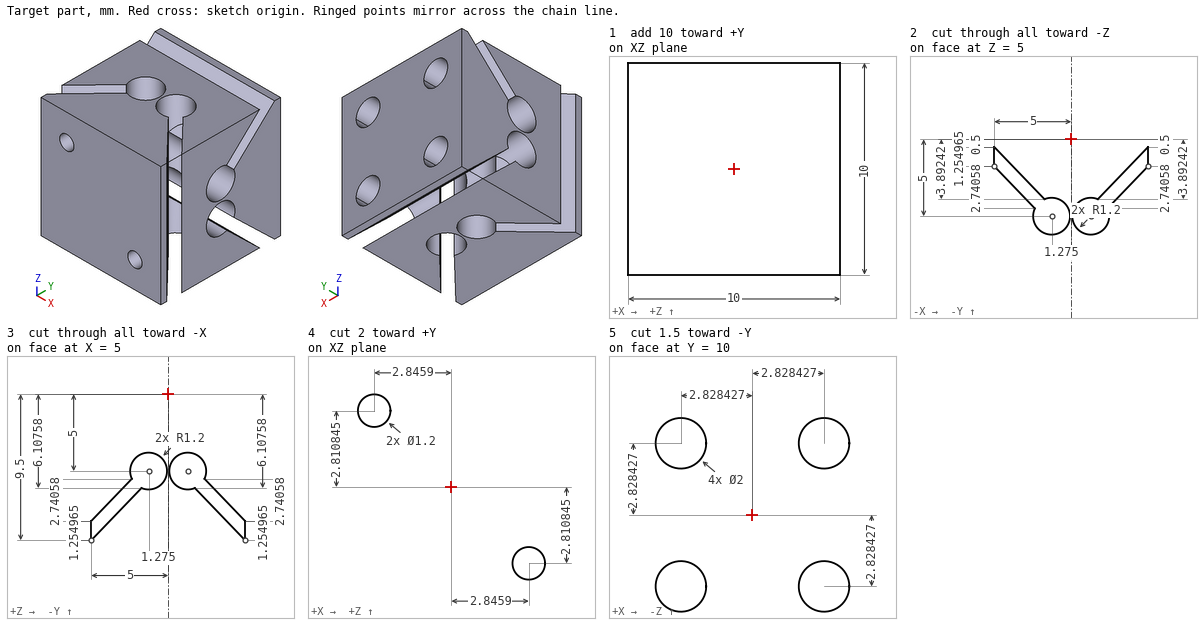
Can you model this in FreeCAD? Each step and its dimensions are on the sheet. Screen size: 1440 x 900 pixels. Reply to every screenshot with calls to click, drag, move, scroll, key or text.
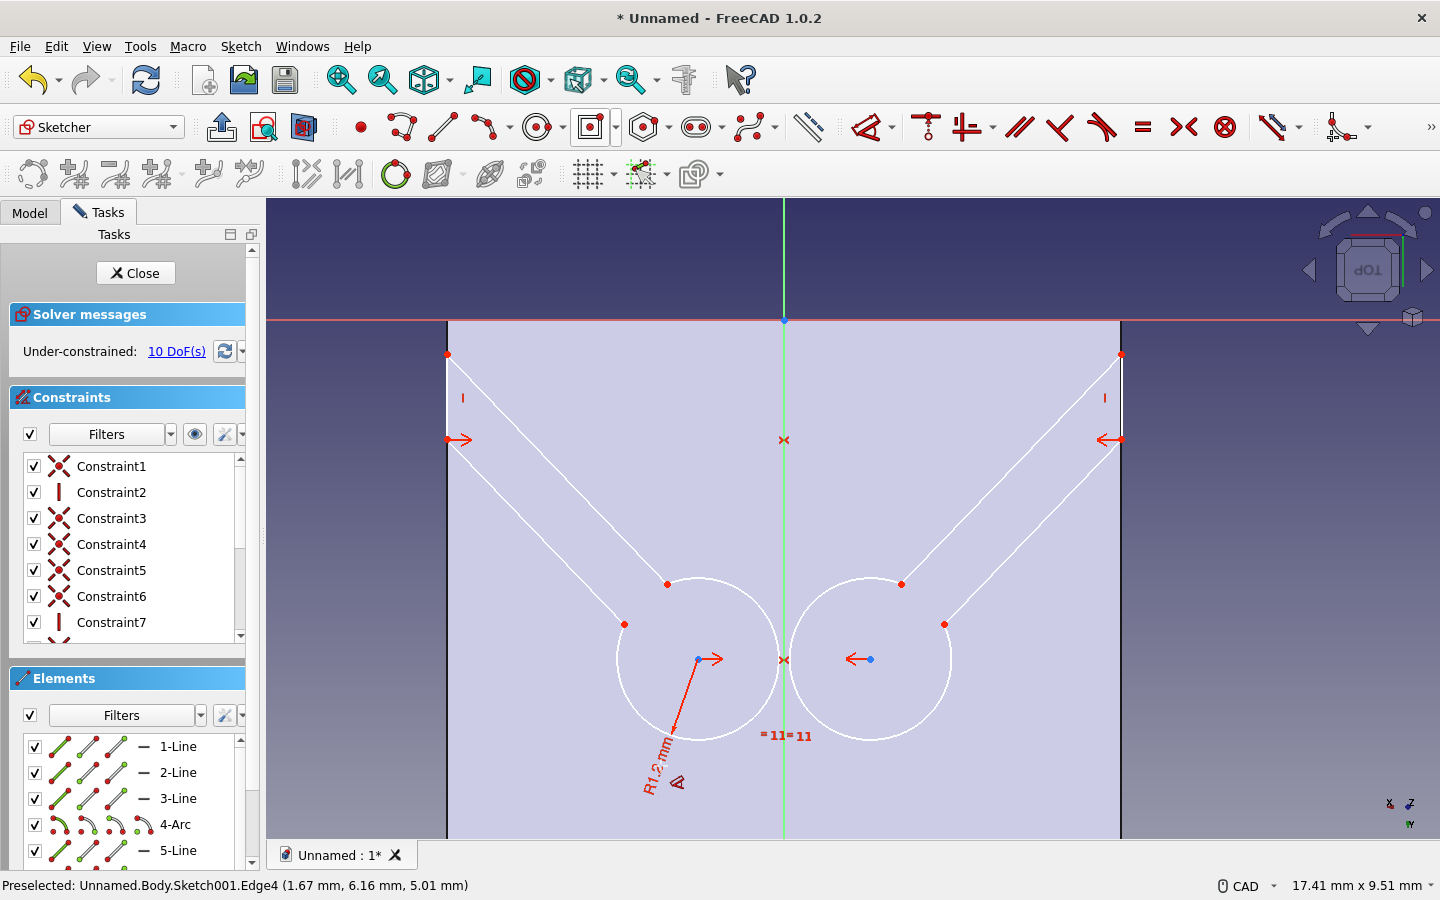
click(447, 355)
click(616, 286)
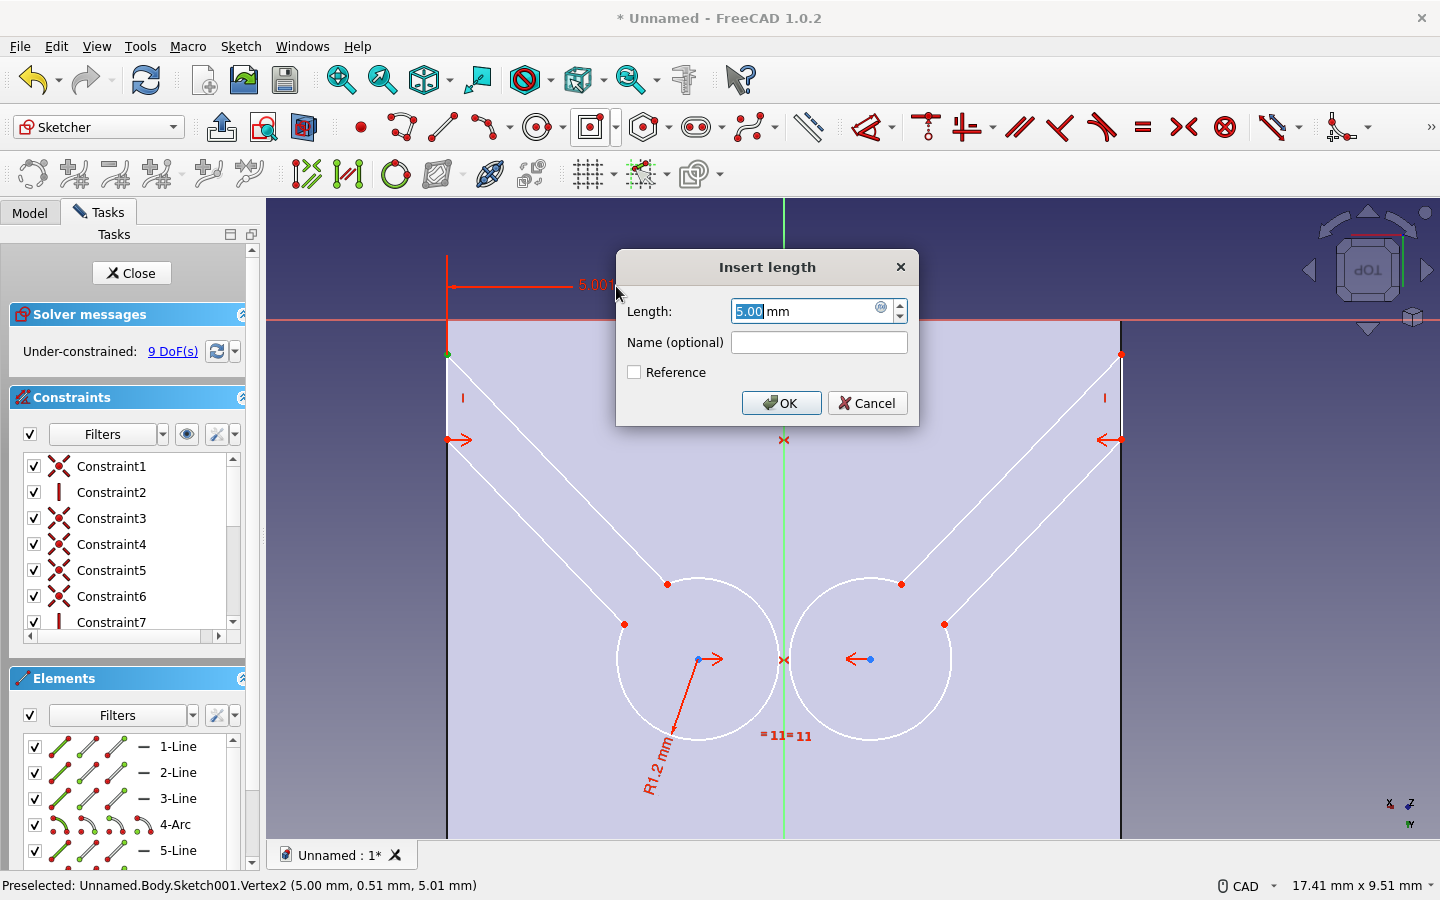
text(5)
key(Return)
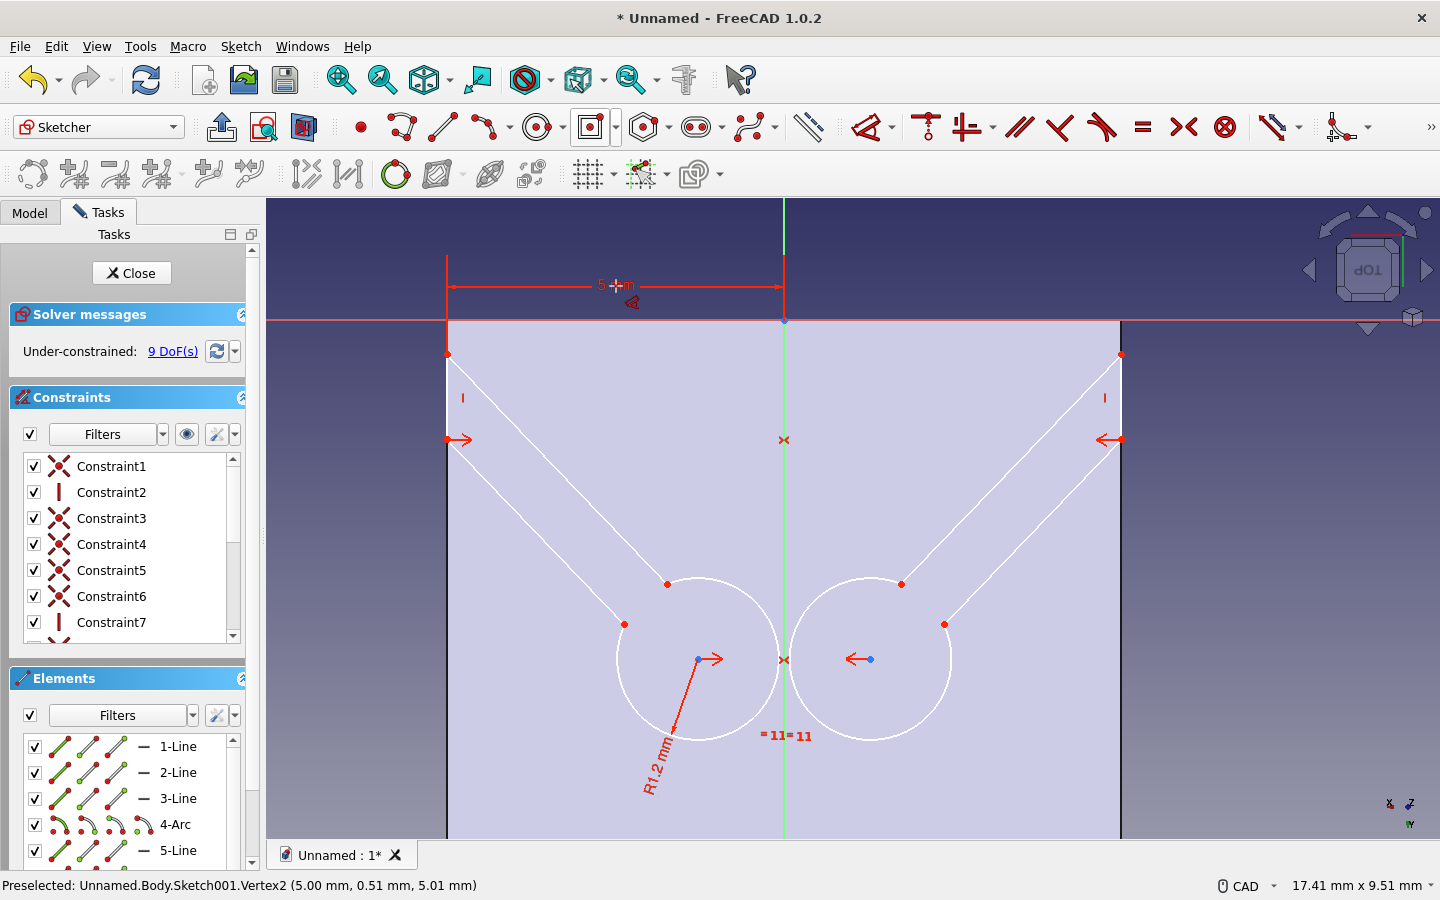
click(698, 659)
click(664, 490)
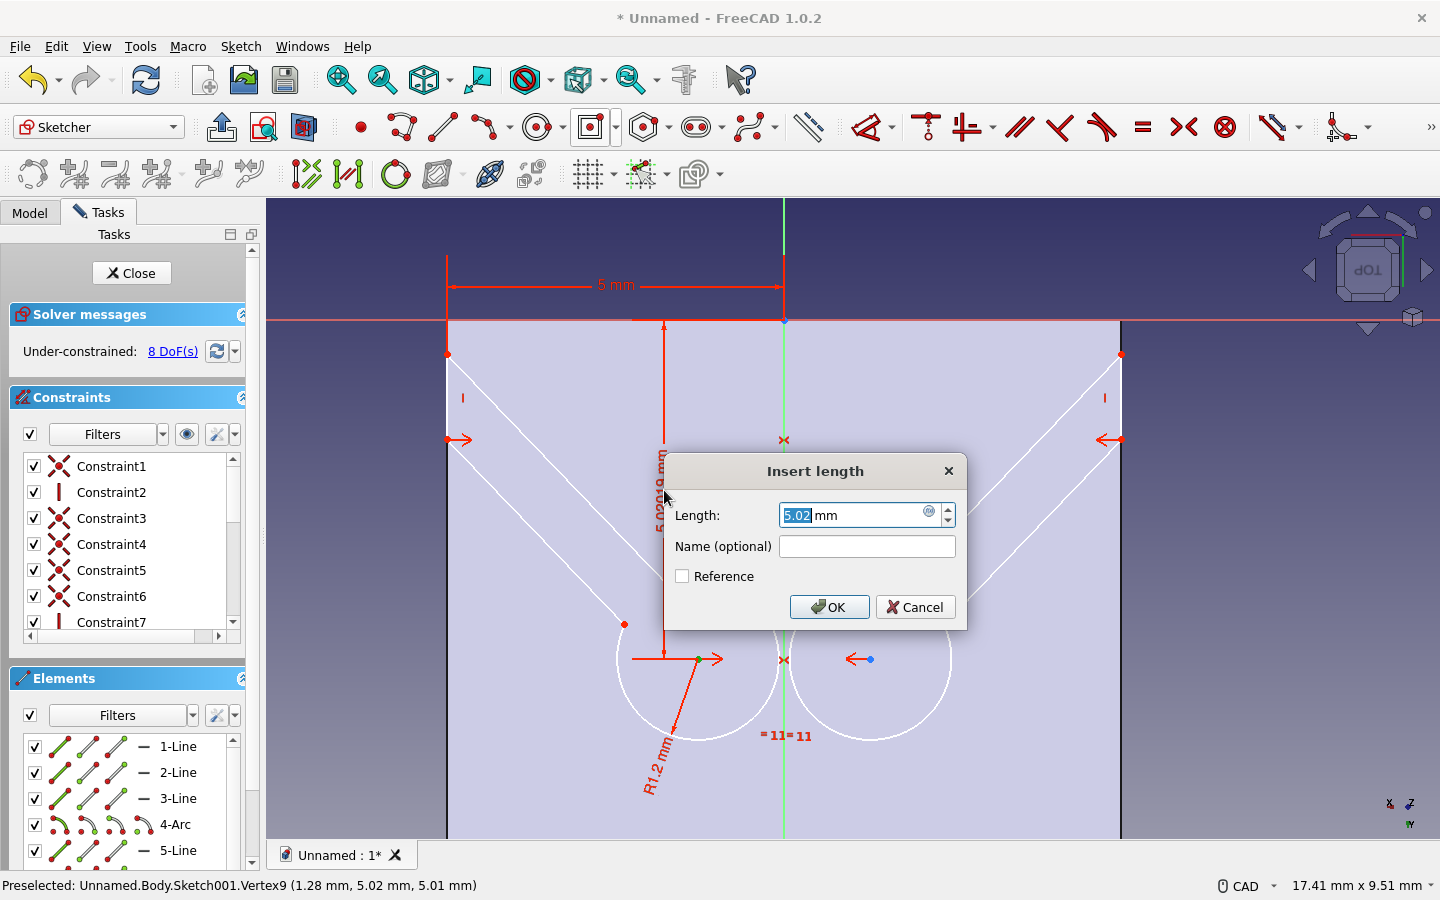
text(5)
key(Return)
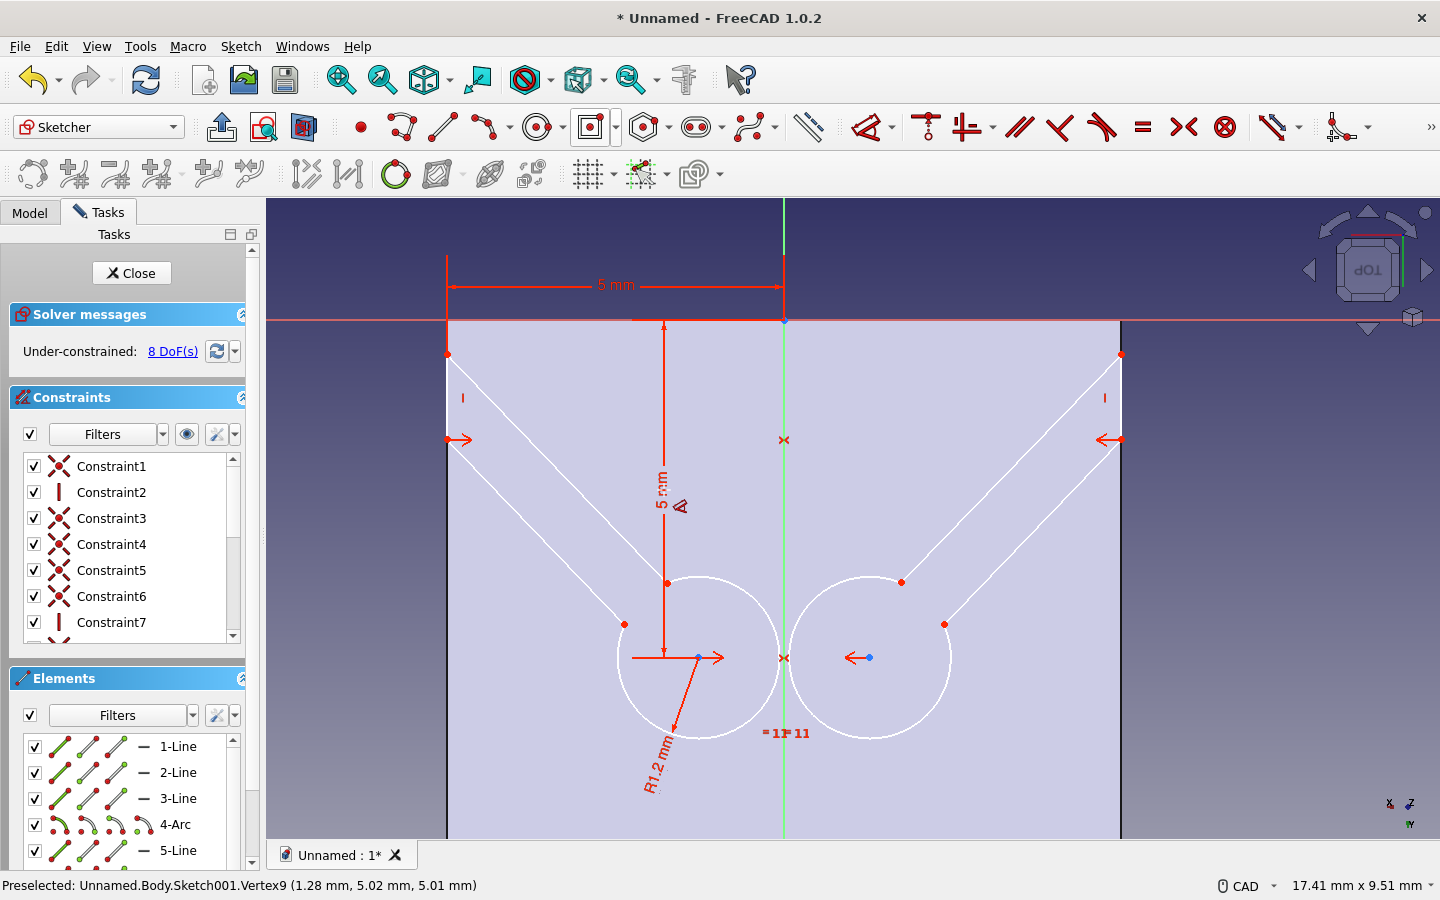
click(447, 355)
click(413, 338)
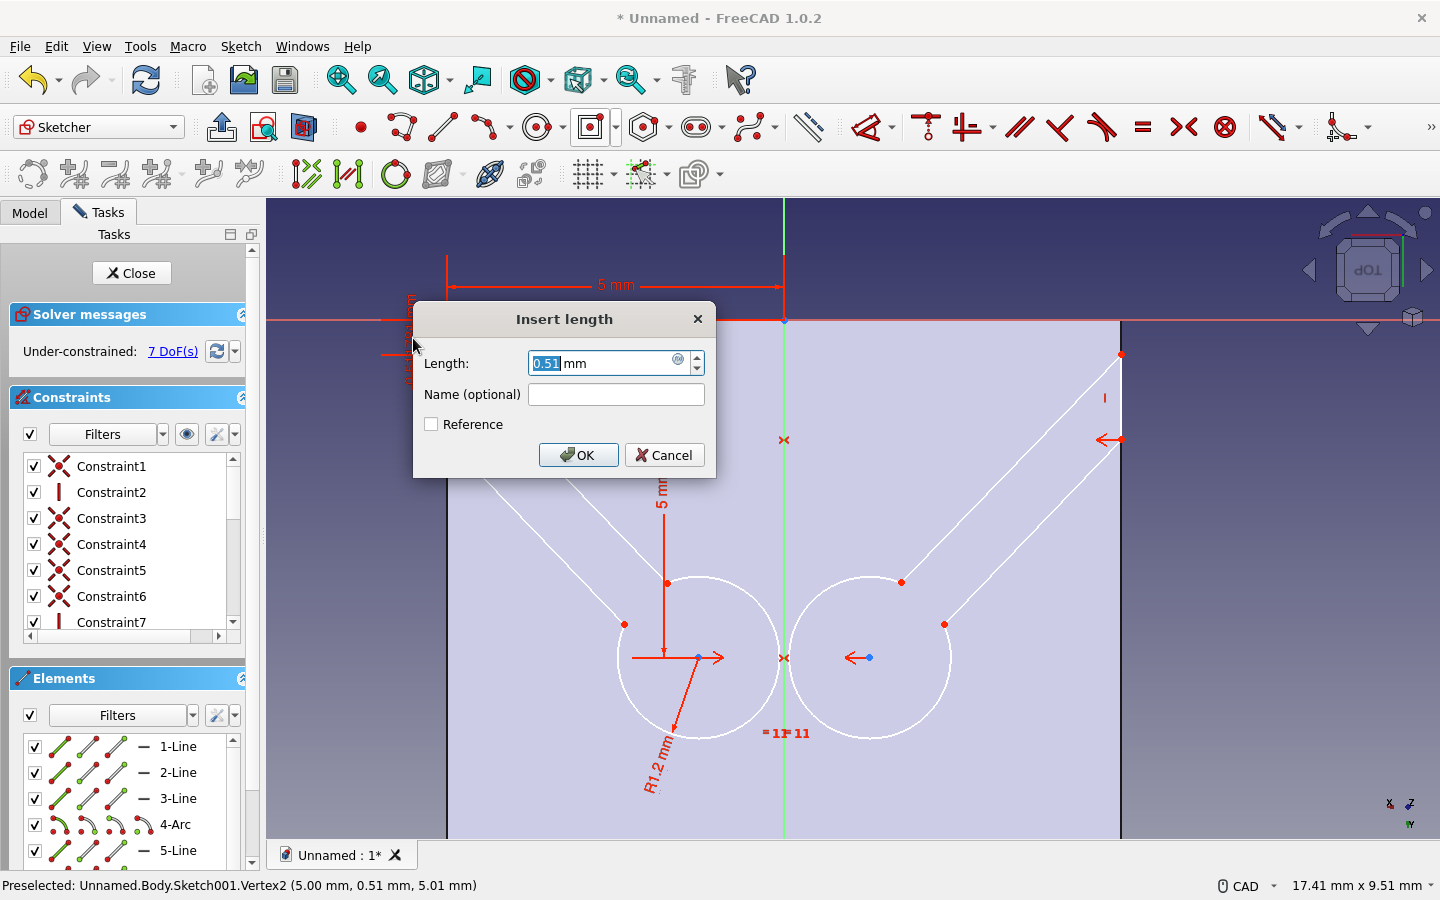
text(0.5)
key(Return)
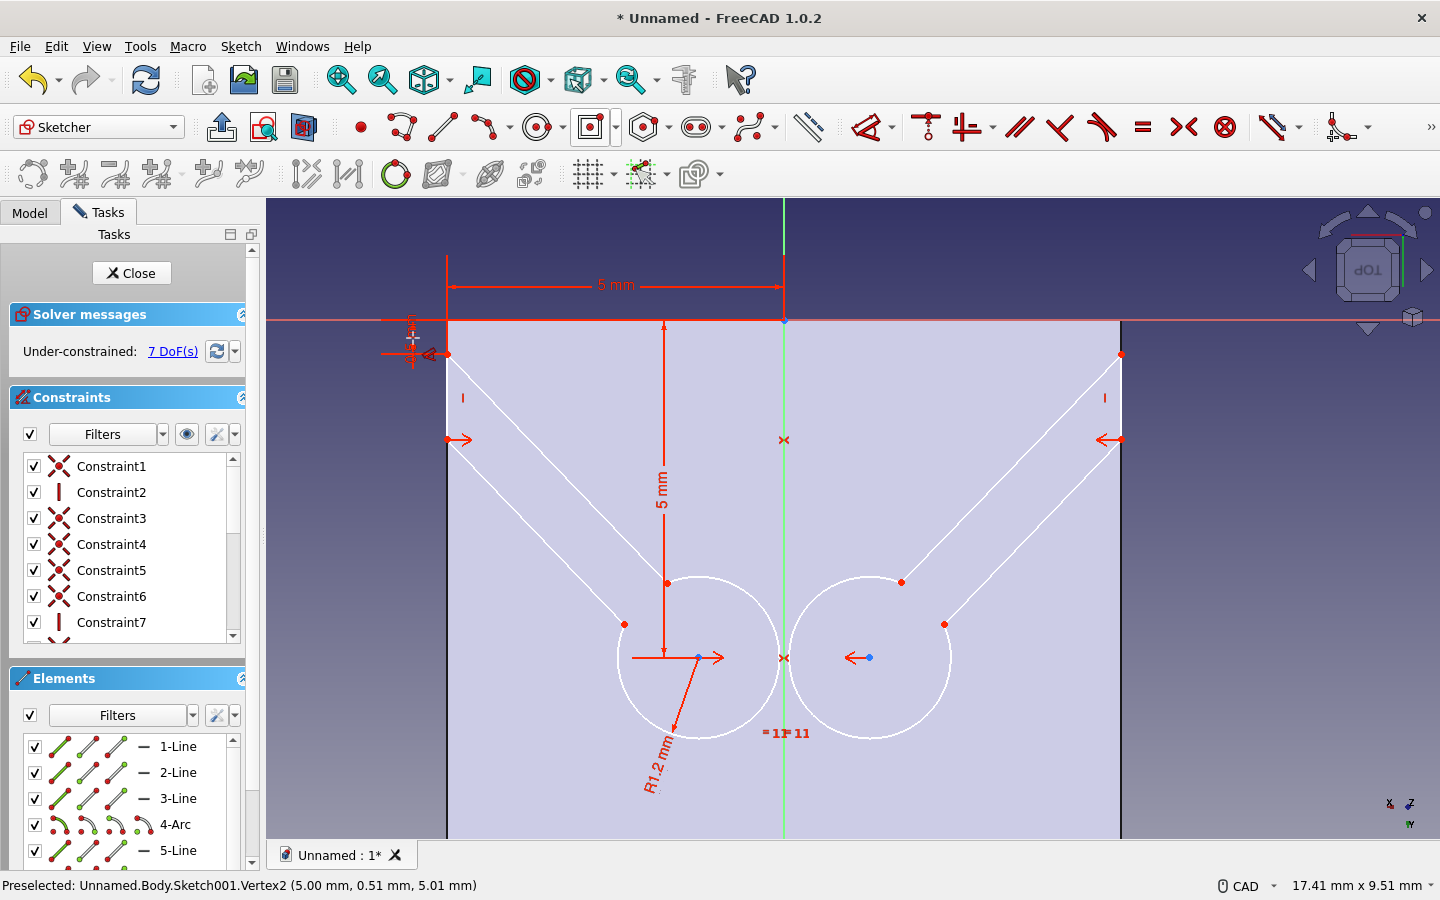
click(1121, 355)
click(1155, 338)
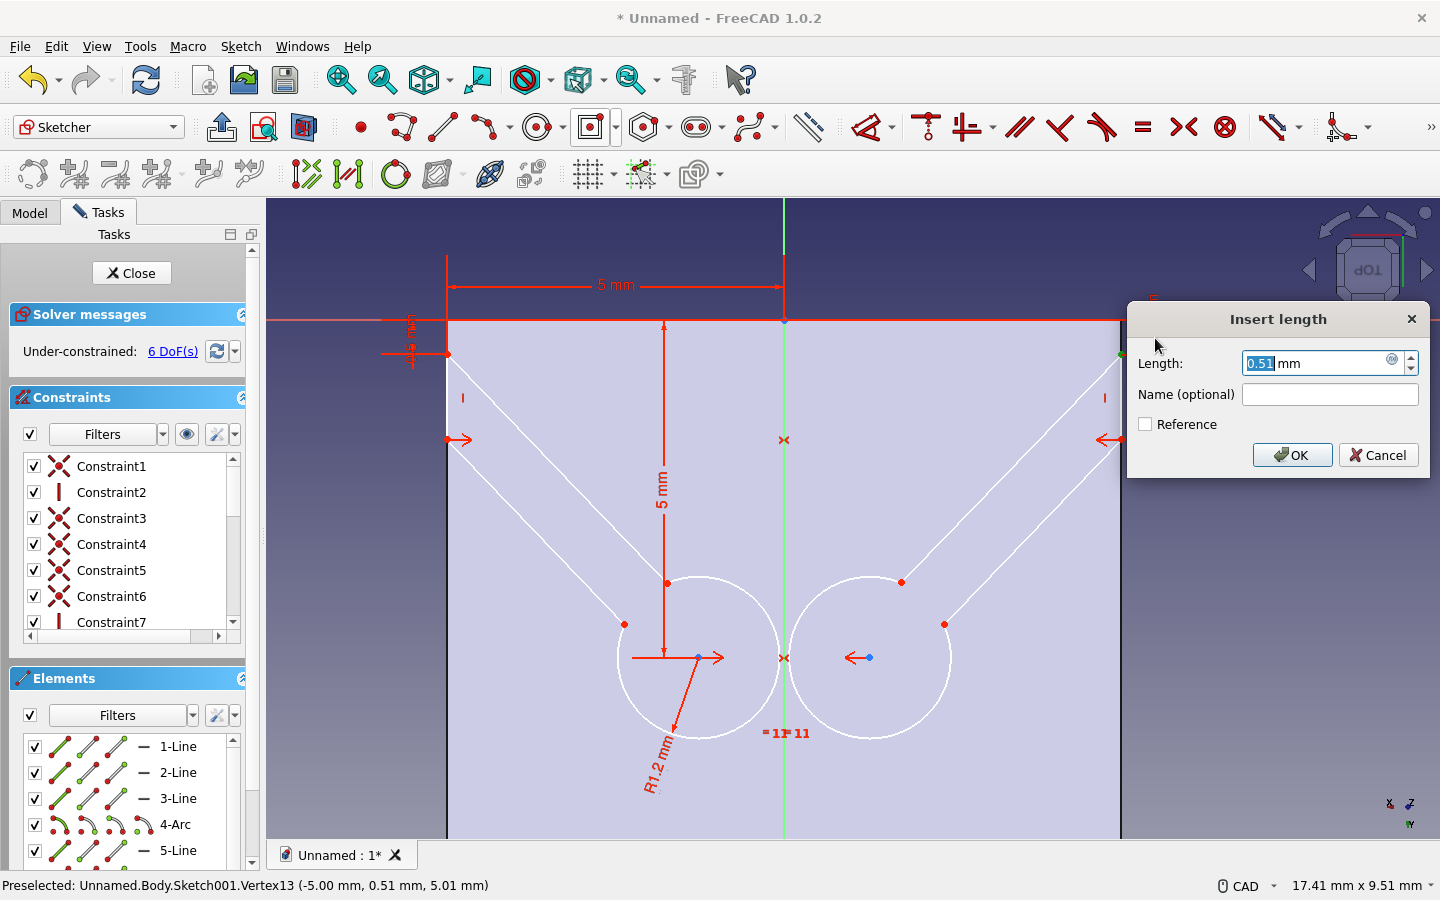
text(0.5)
key(Return)